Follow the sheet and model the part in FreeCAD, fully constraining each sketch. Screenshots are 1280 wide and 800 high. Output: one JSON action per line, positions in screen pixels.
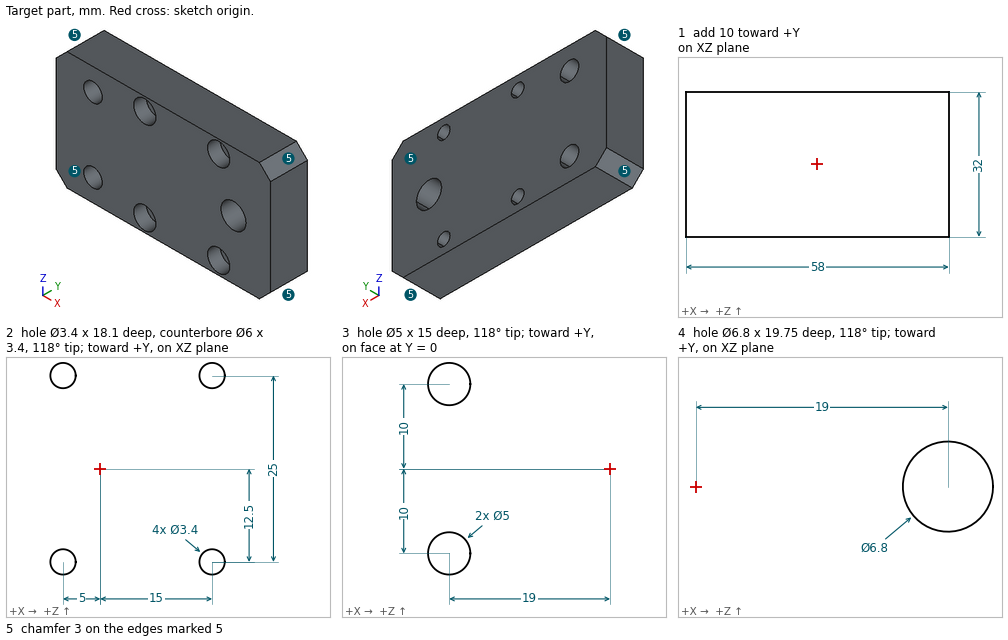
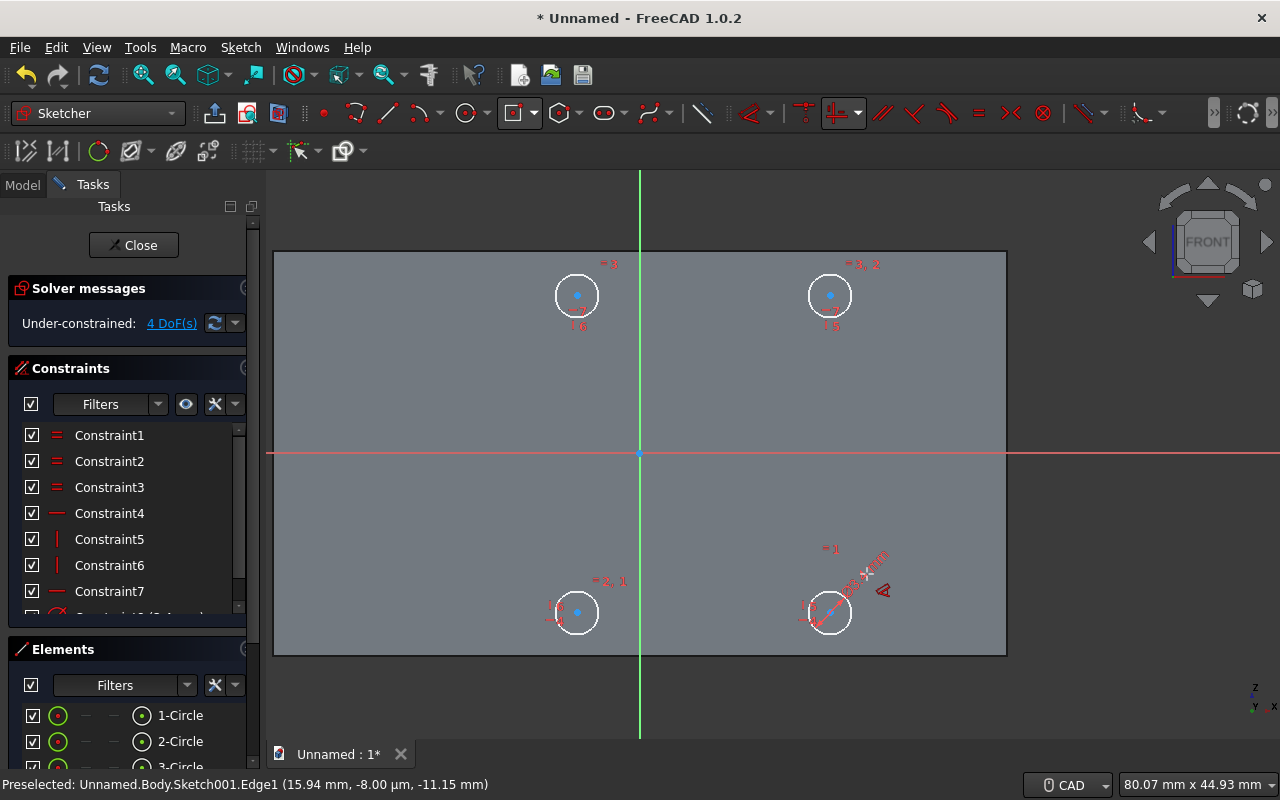
{"action": "left_click", "coordinate": [577, 613]}
{"action": "left_click", "coordinate": [608, 647]}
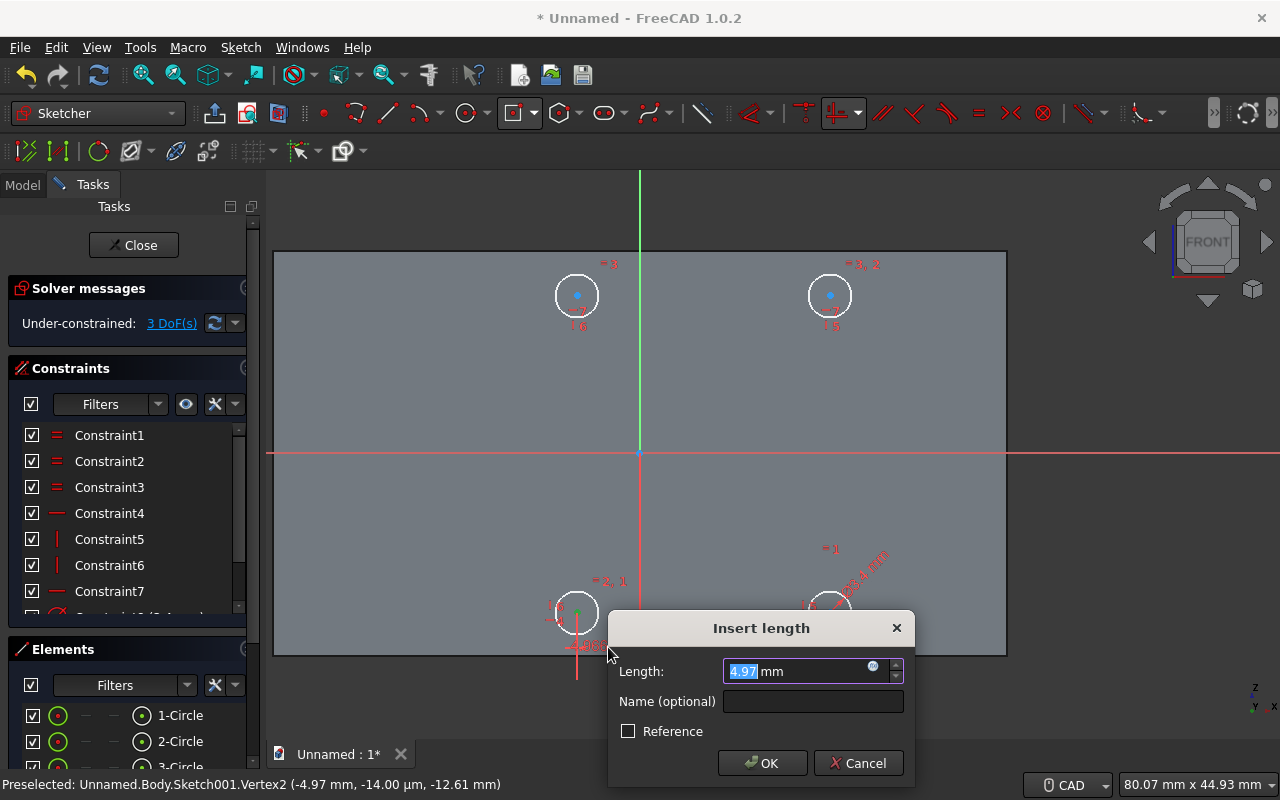
{"action": "type", "text": "5"}
{"action": "key", "text": "Return"}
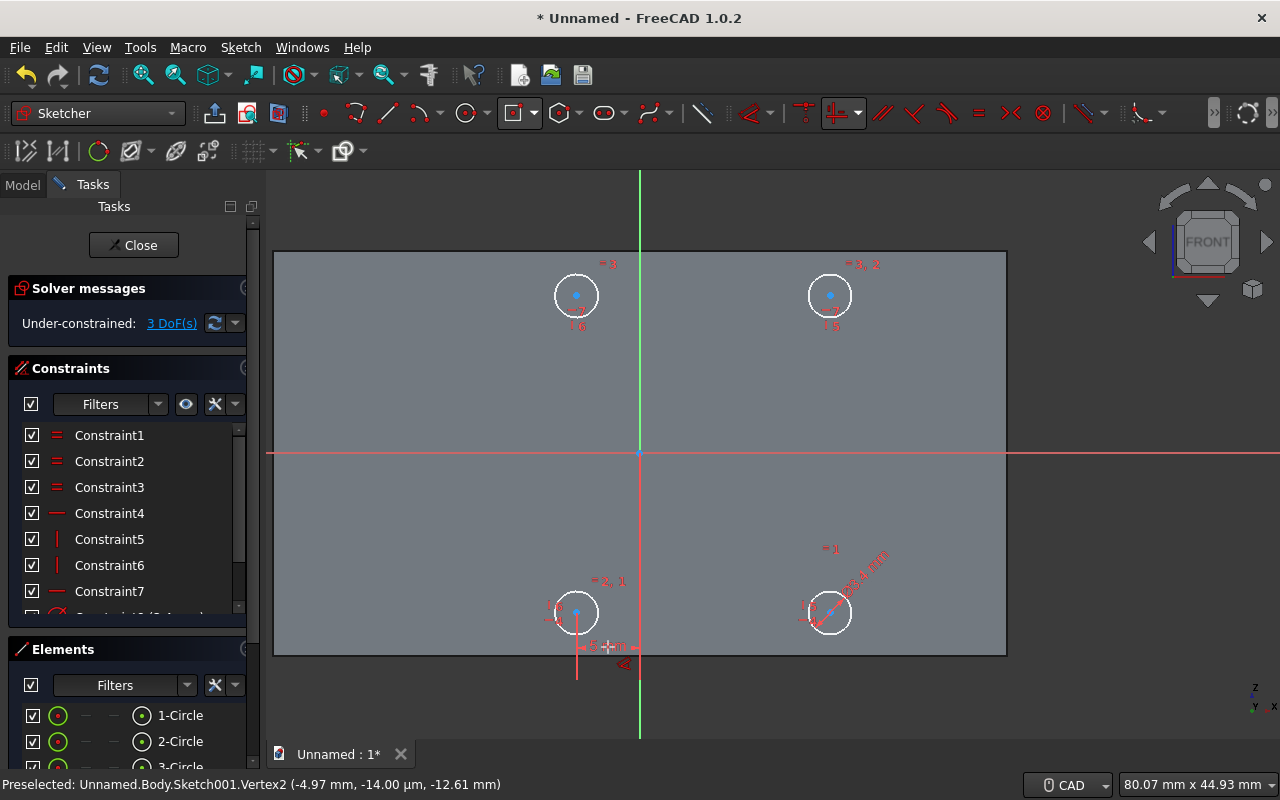
{"action": "left_click", "coordinate": [830, 613]}
{"action": "left_click", "coordinate": [735, 647]}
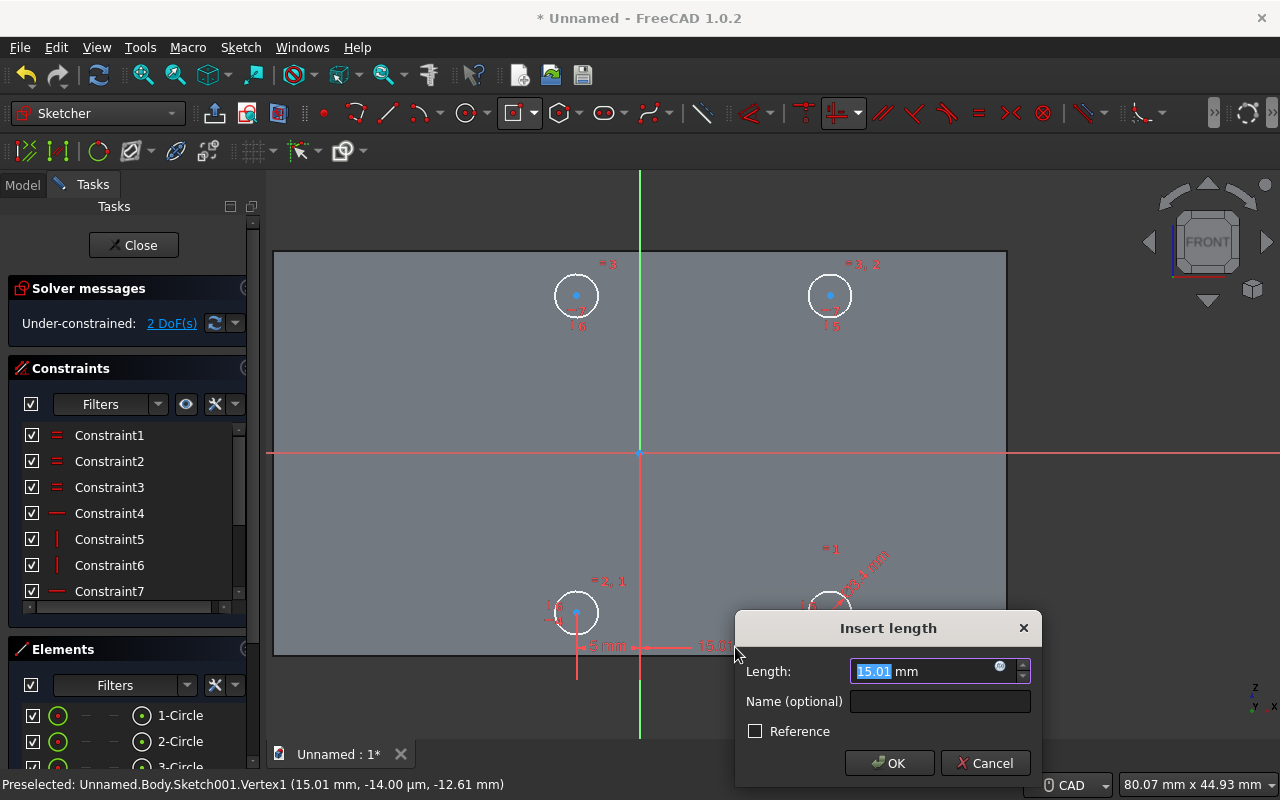
{"action": "type", "text": "15"}
{"action": "key", "text": "Return"}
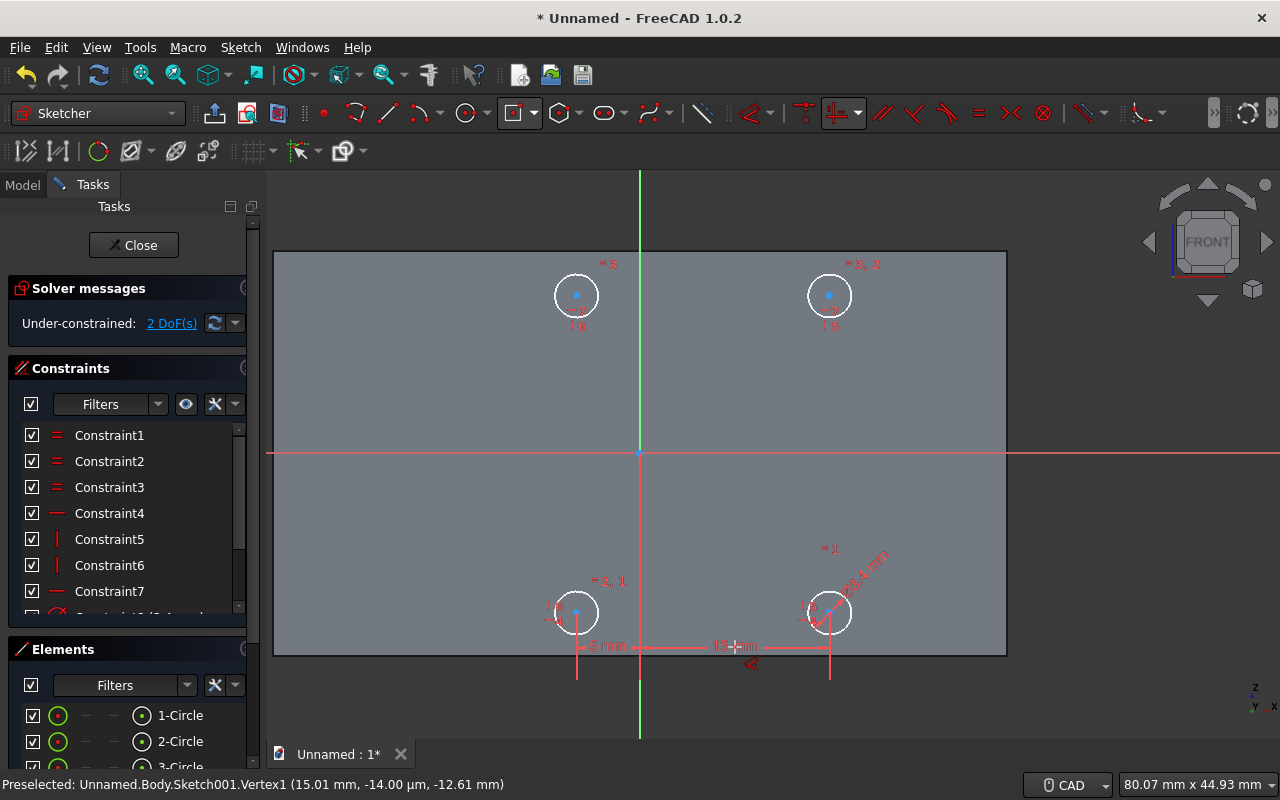
{"action": "left_click", "coordinate": [830, 613]}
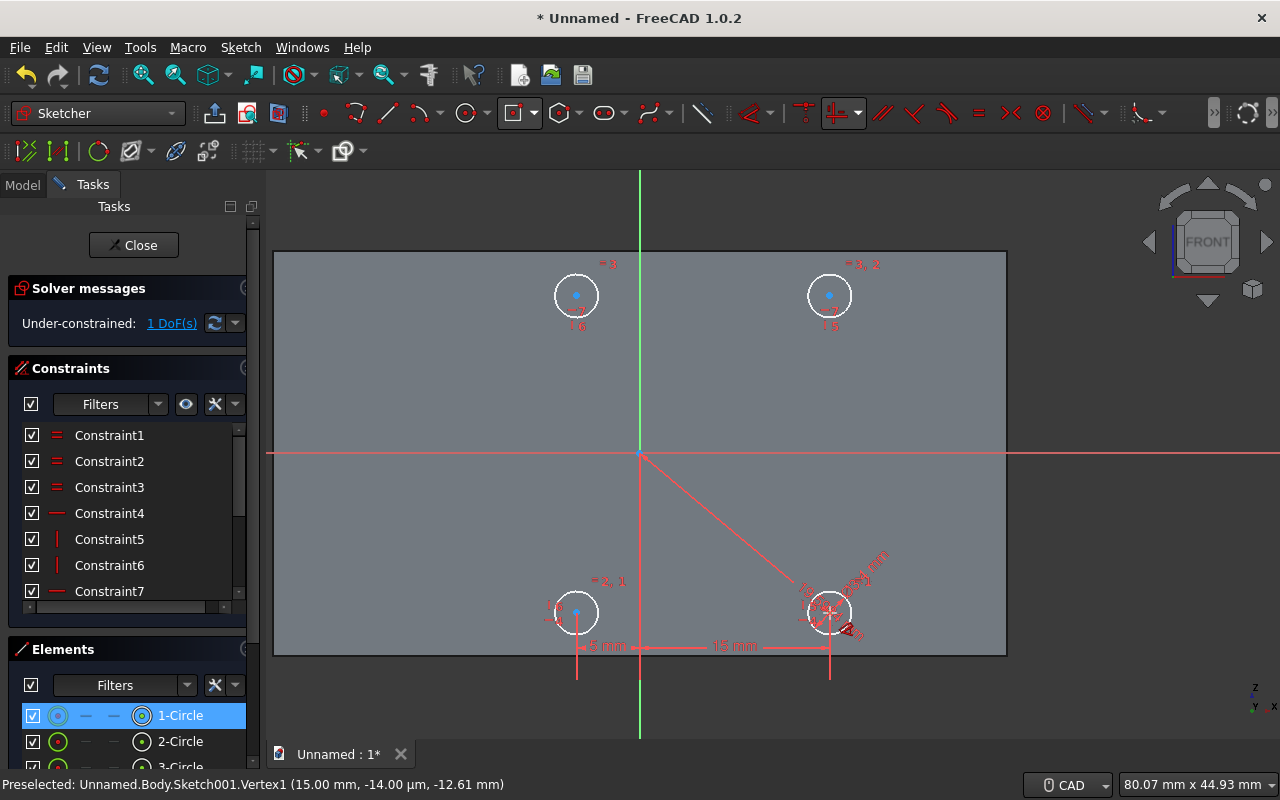
{"action": "left_click", "coordinate": [830, 296]}
{"action": "left_click", "coordinate": [864, 382]}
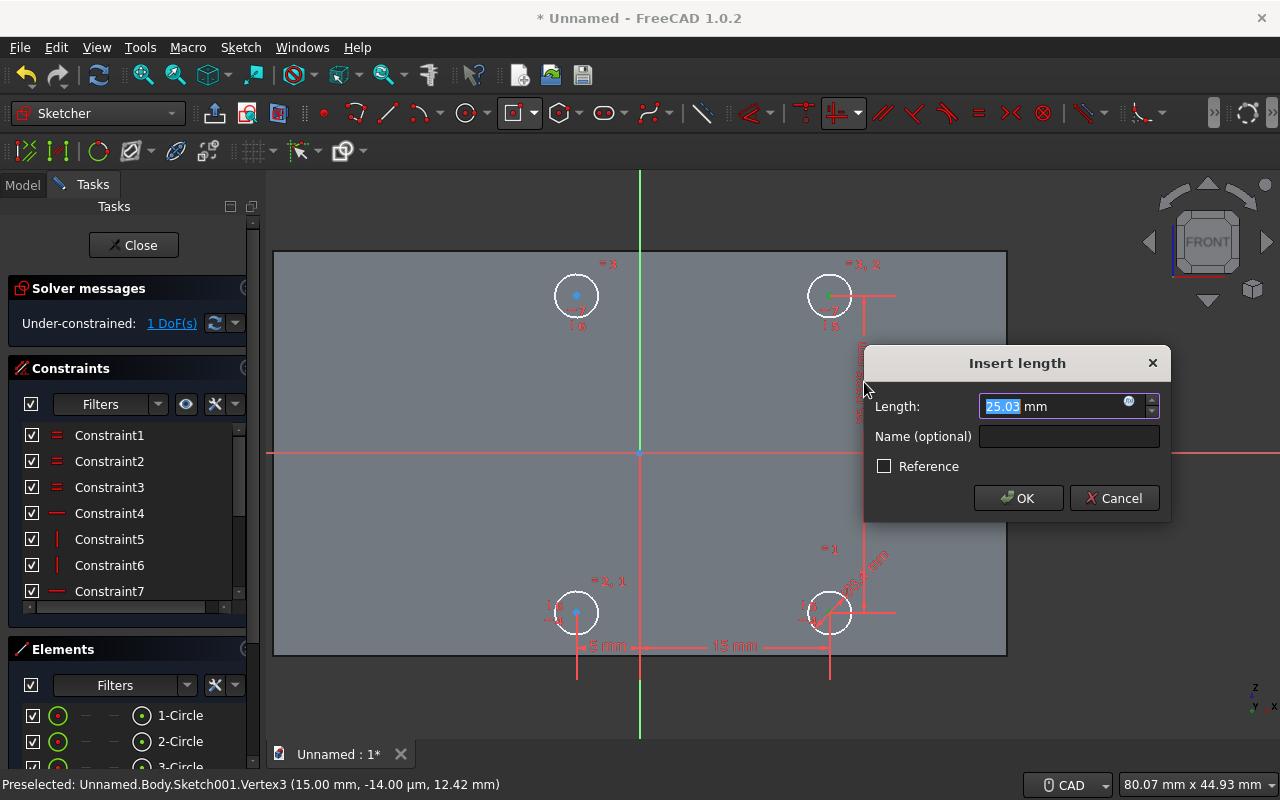
{"action": "type", "text": "25"}
{"action": "key", "text": "Return"}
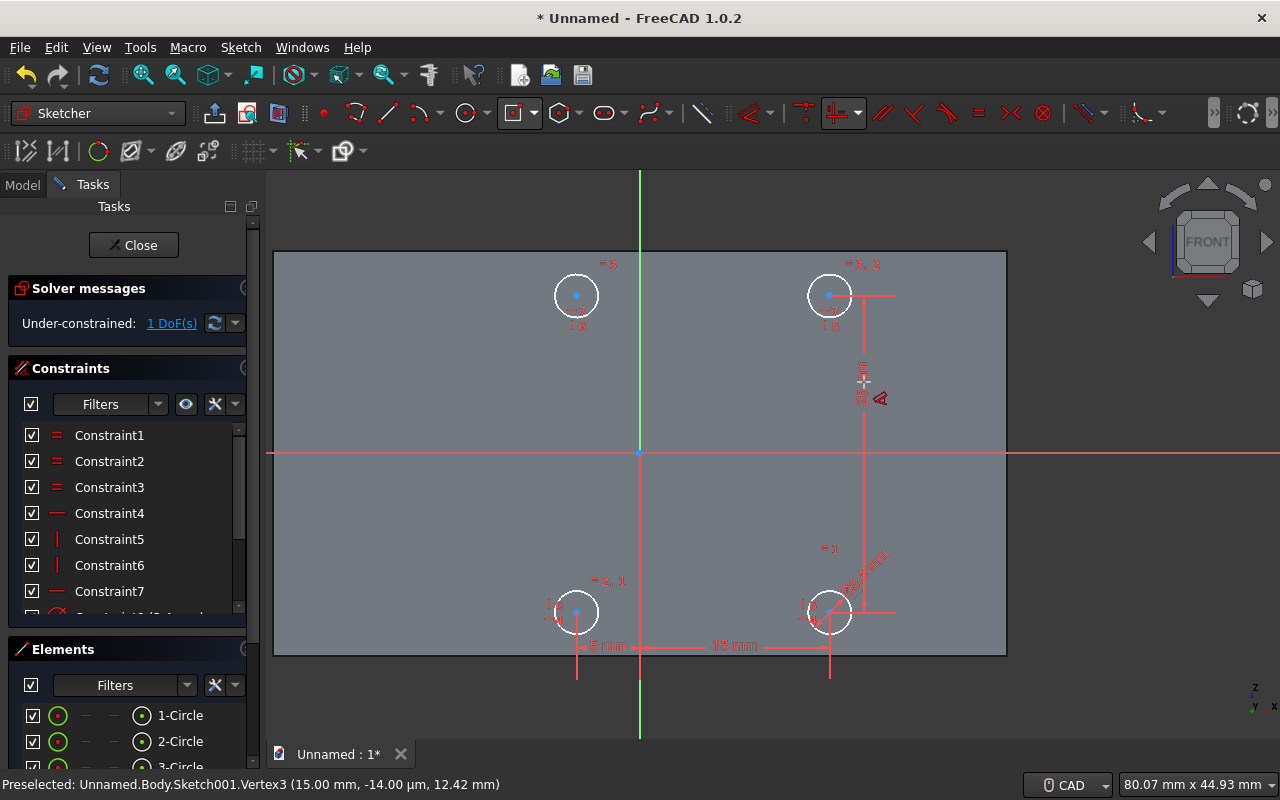
{"action": "left_click", "coordinate": [830, 613]}
{"action": "left_click", "coordinate": [864, 533]}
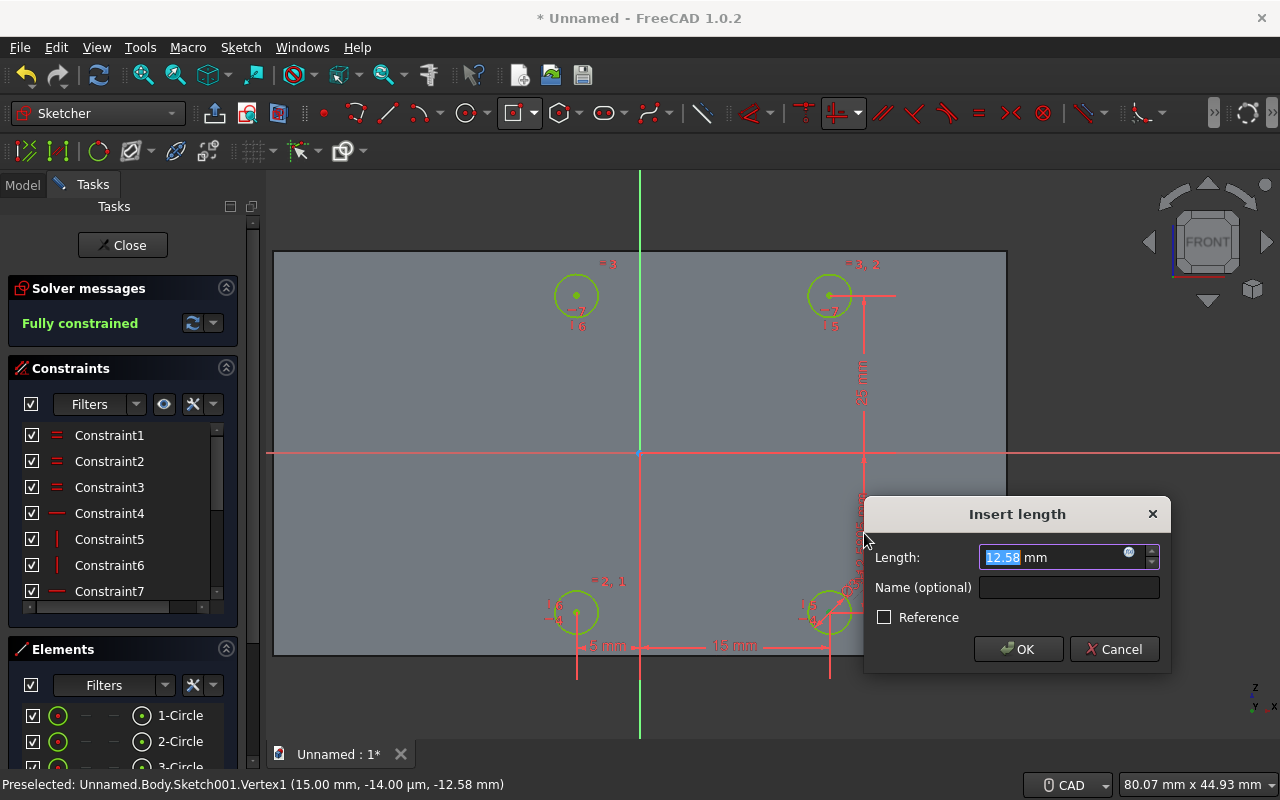
{"action": "type", "text": "12.5"}
{"action": "key", "text": "Return"}
{"action": "key", "text": "Escape"}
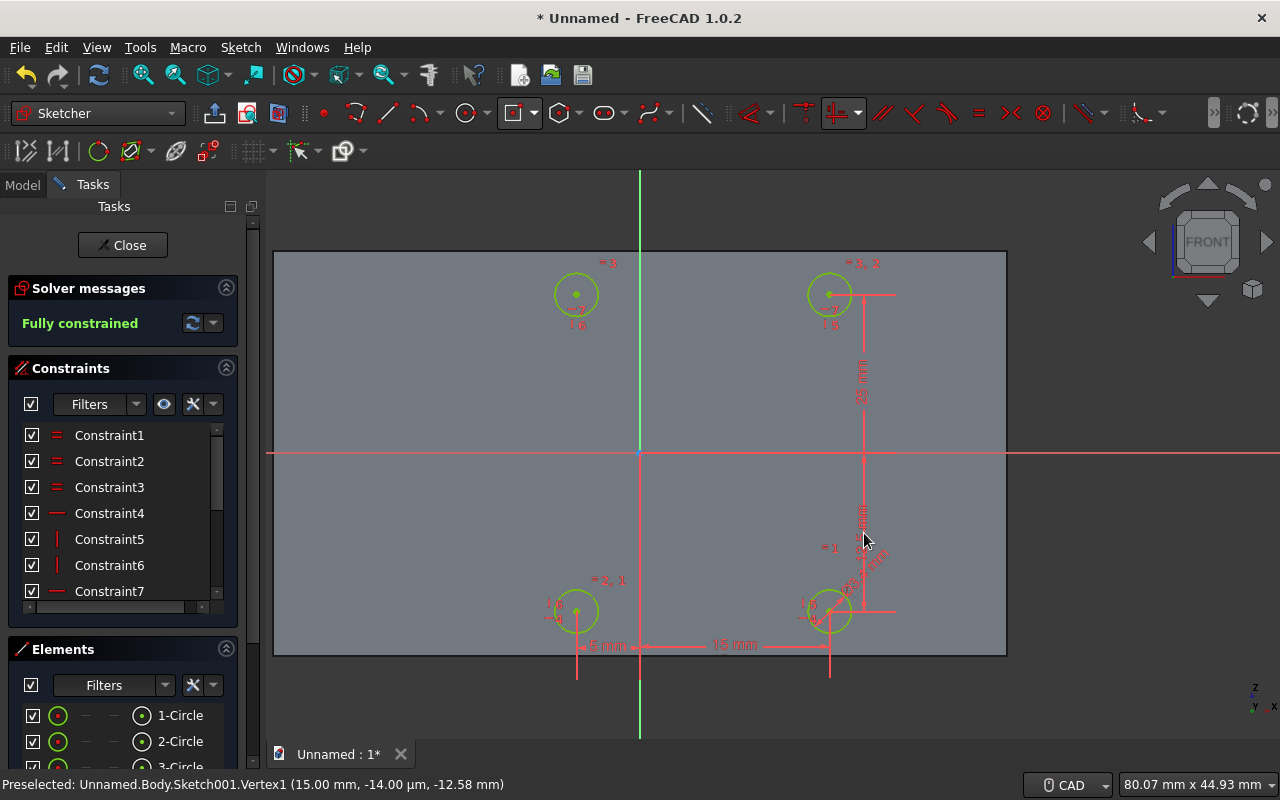
{"action": "left_click", "coordinate": [123, 245]}